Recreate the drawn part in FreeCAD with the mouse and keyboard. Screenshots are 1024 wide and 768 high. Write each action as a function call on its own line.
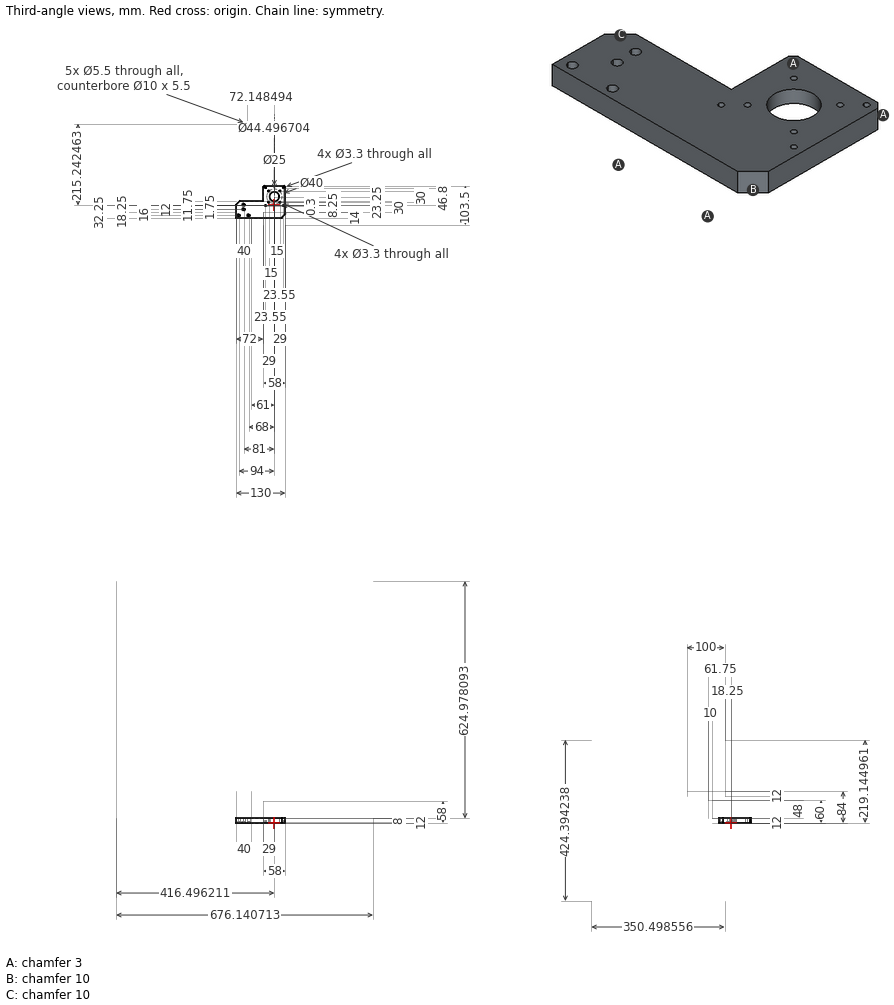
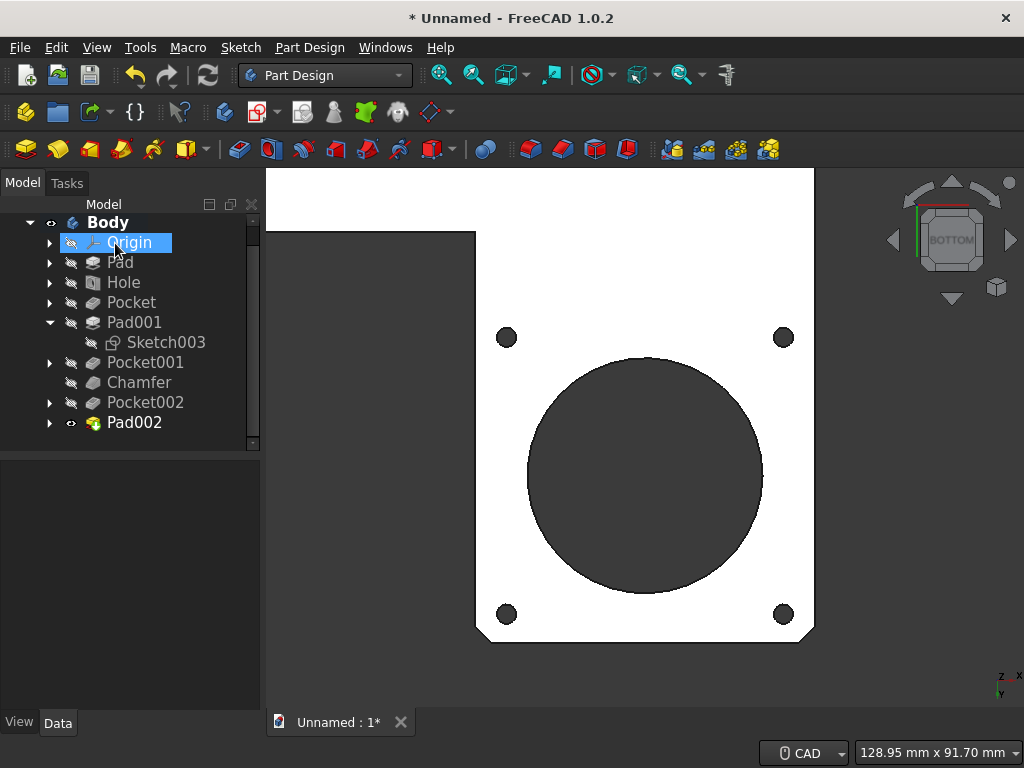
click(442, 76)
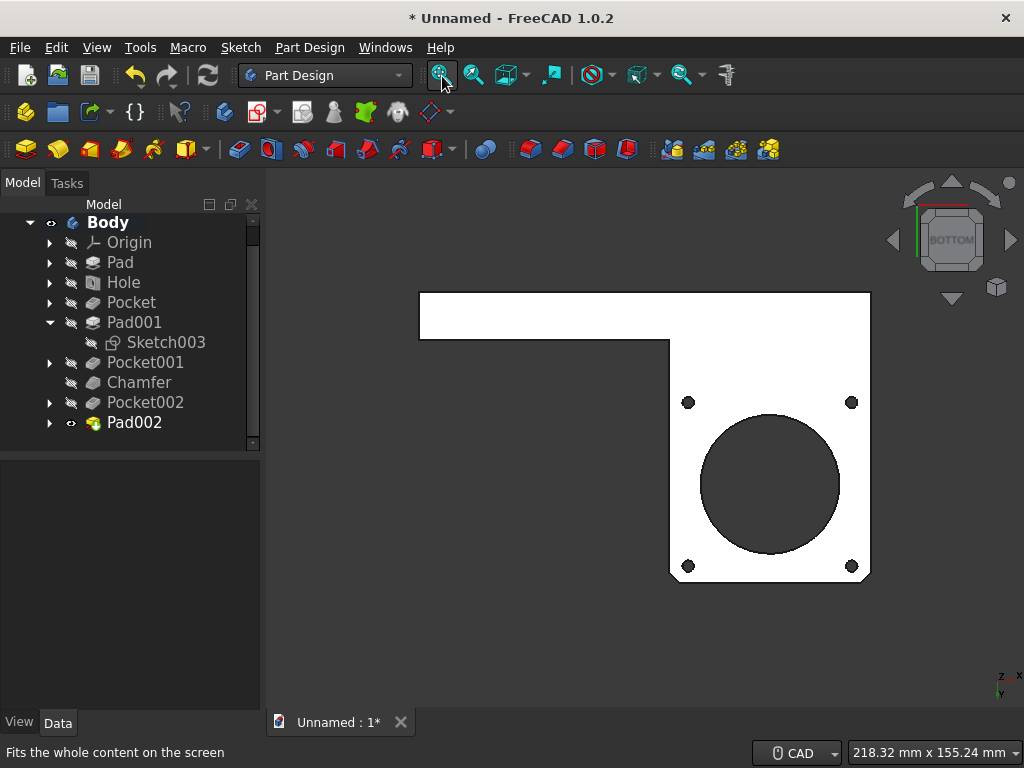
key(0)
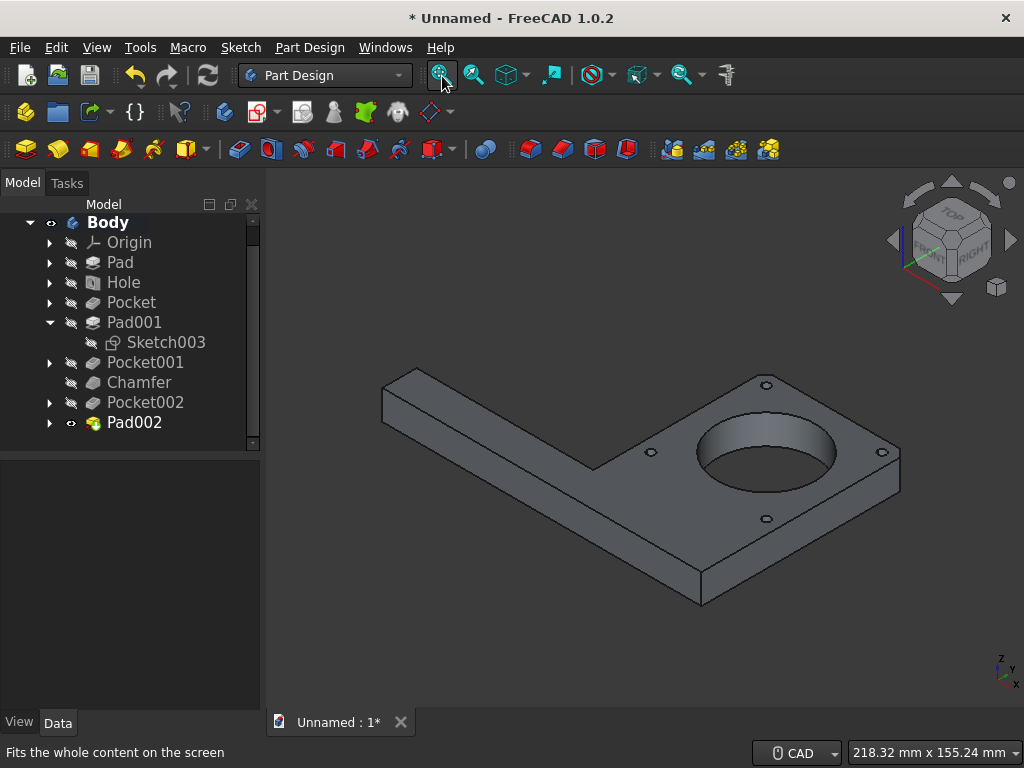
click(677, 506)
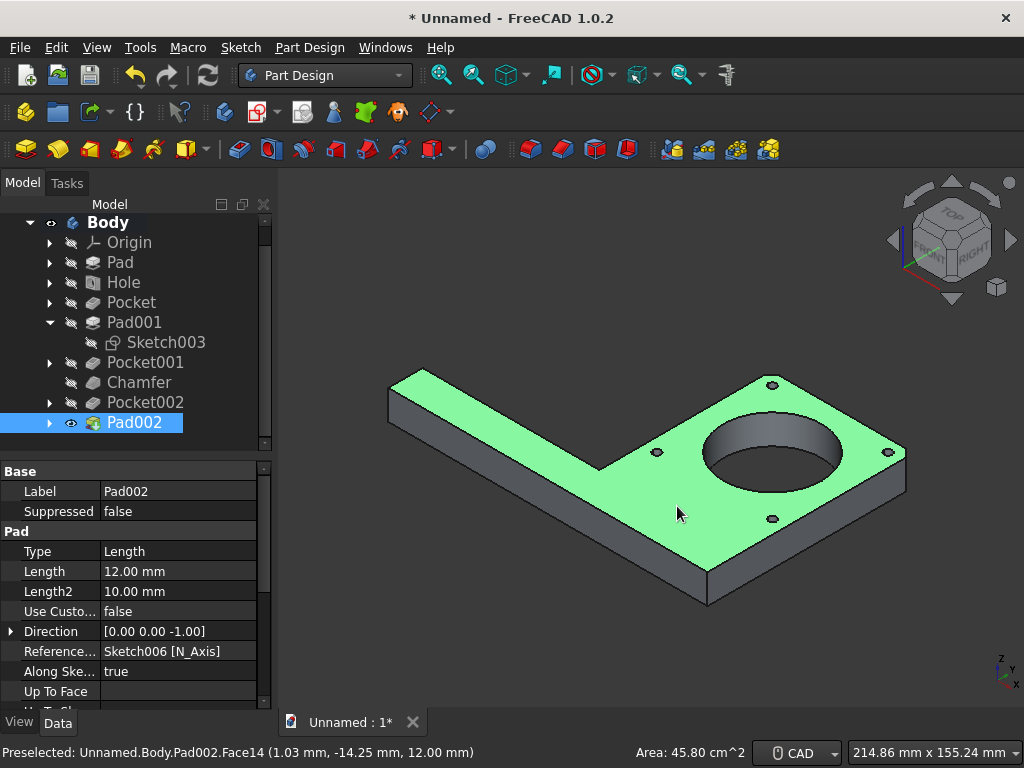
click(258, 112)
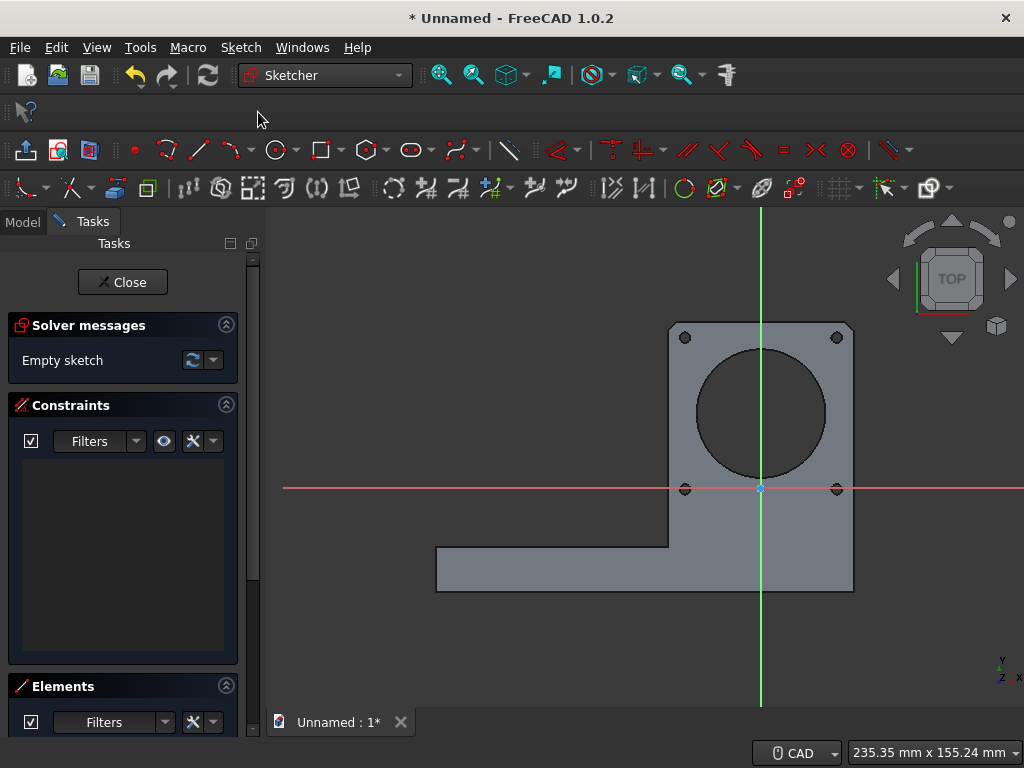
scroll(467, 618, up, 6)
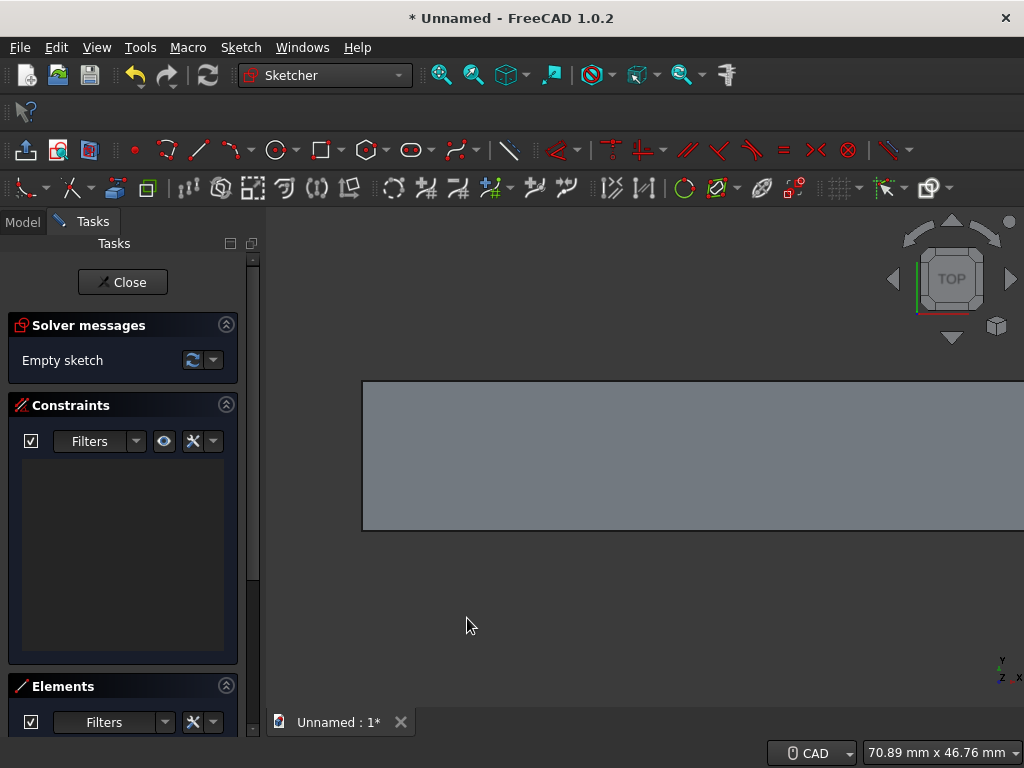
key(g)
key(r)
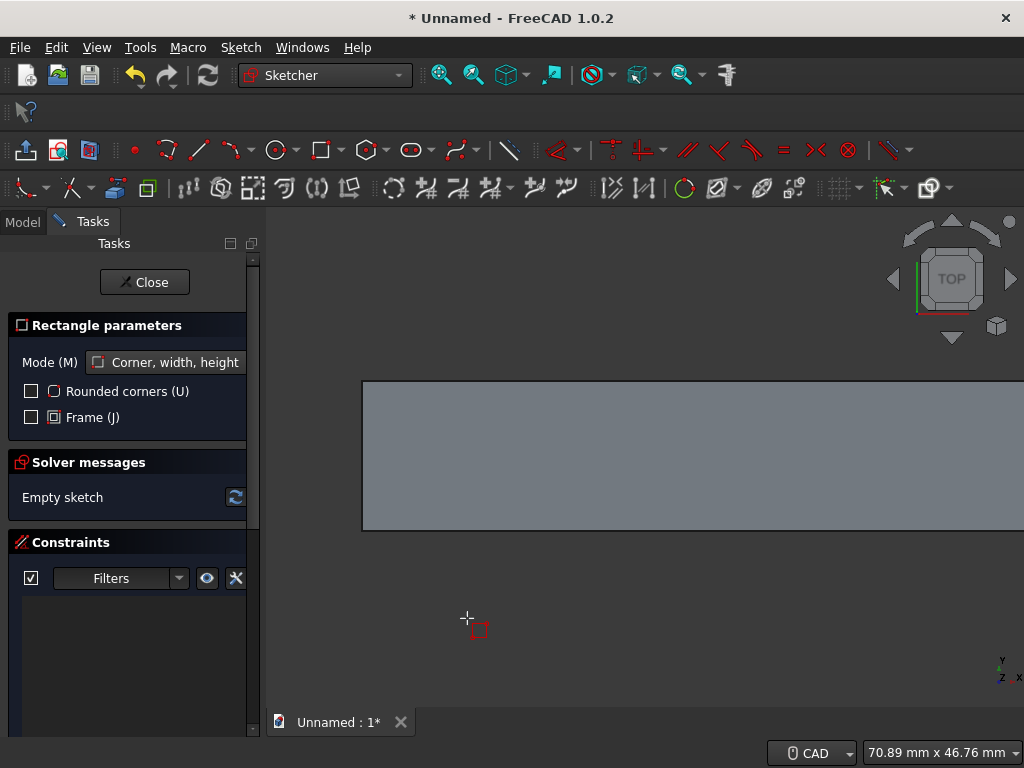
click(362, 381)
move(790, 531)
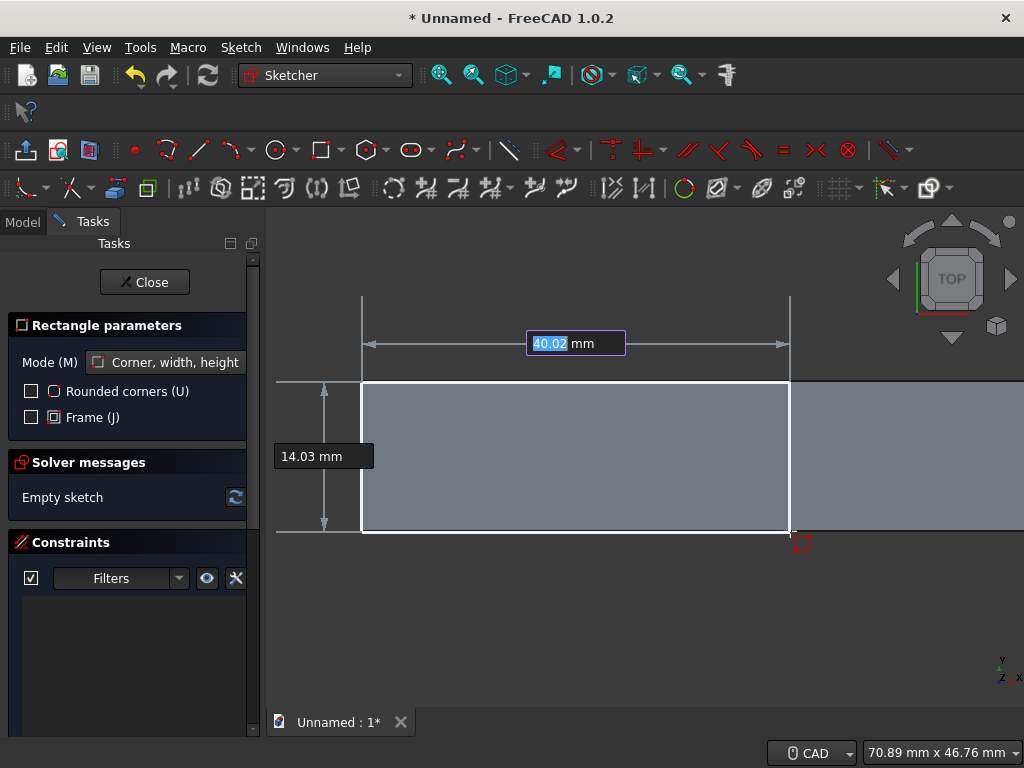
text(40)
key(Tab)
text(14)
key(Return)
key(Escape)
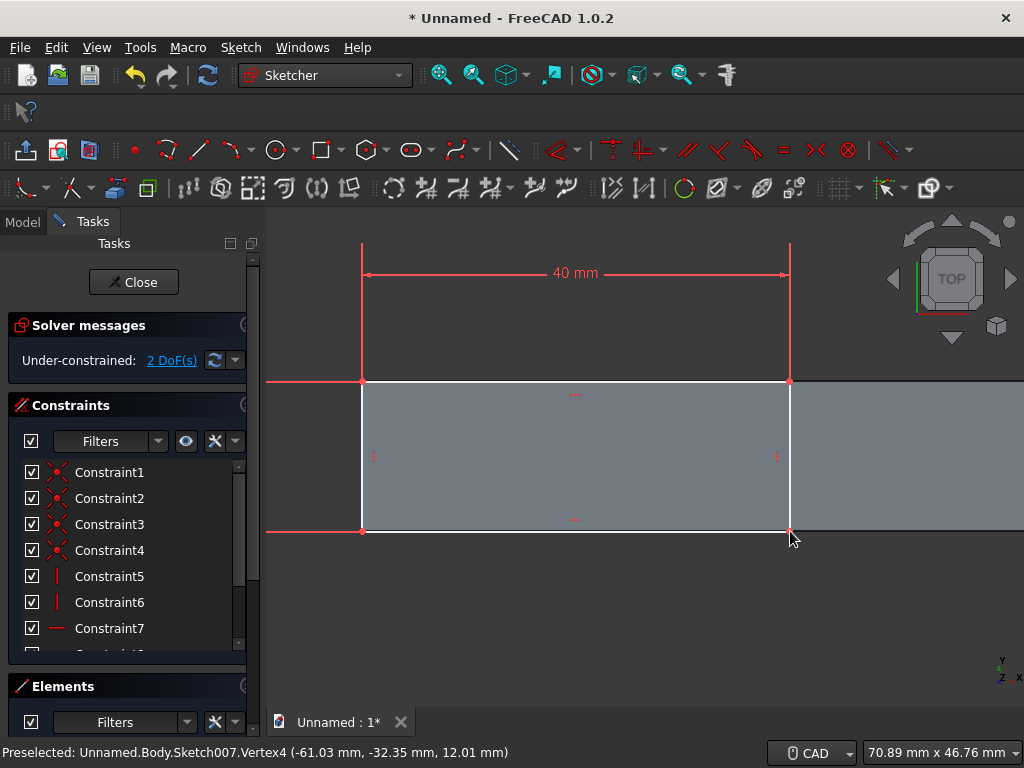
click(556, 150)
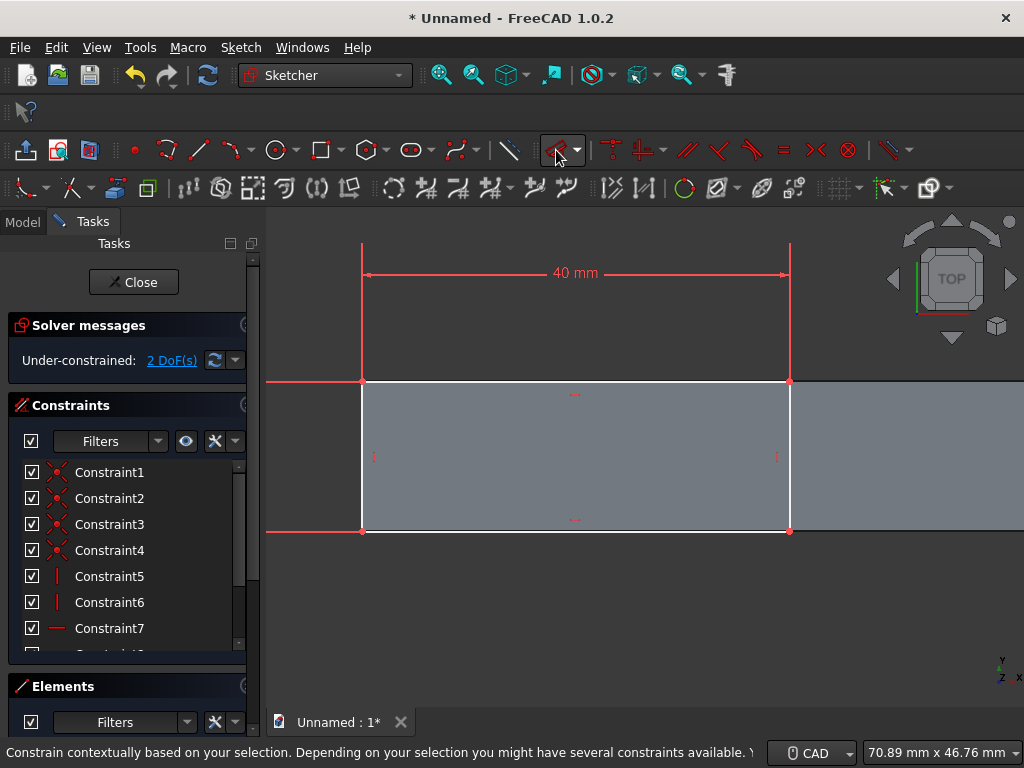
click(790, 532)
click(824, 566)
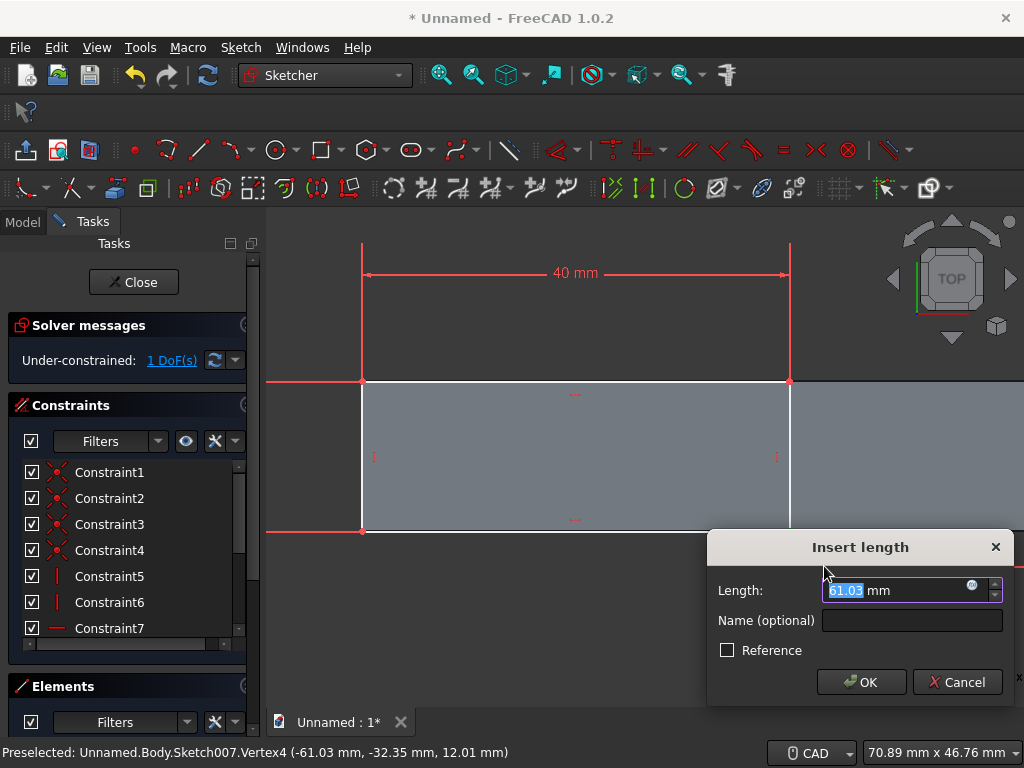
text(61)
key(Return)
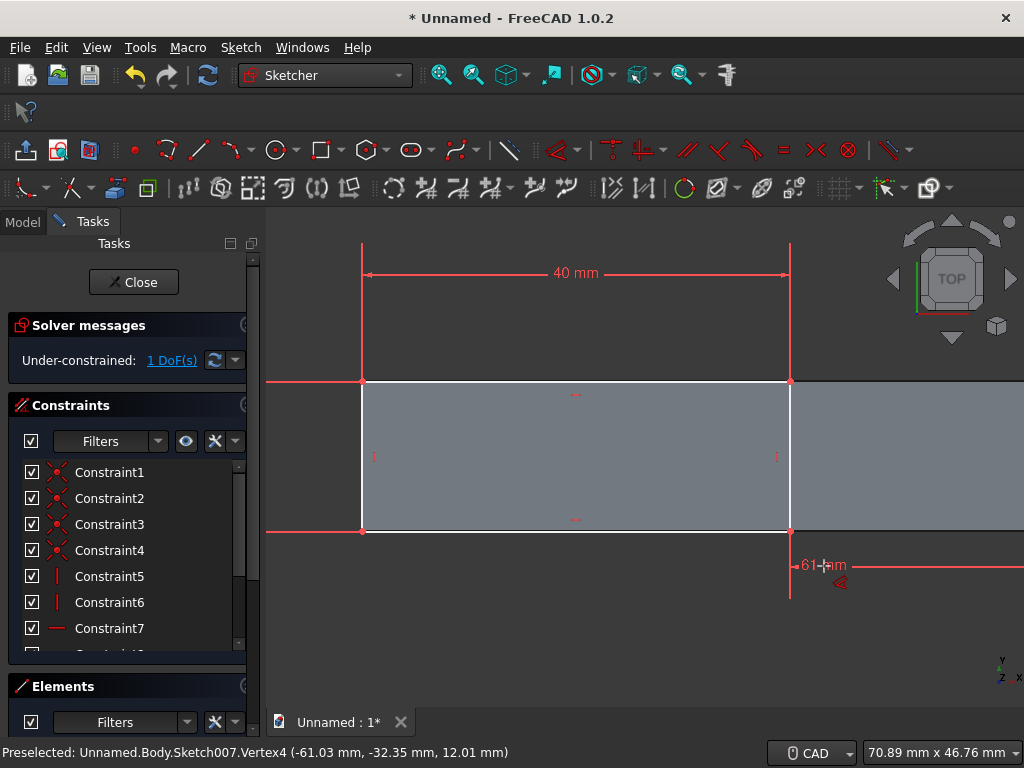
click(362, 382)
click(328, 309)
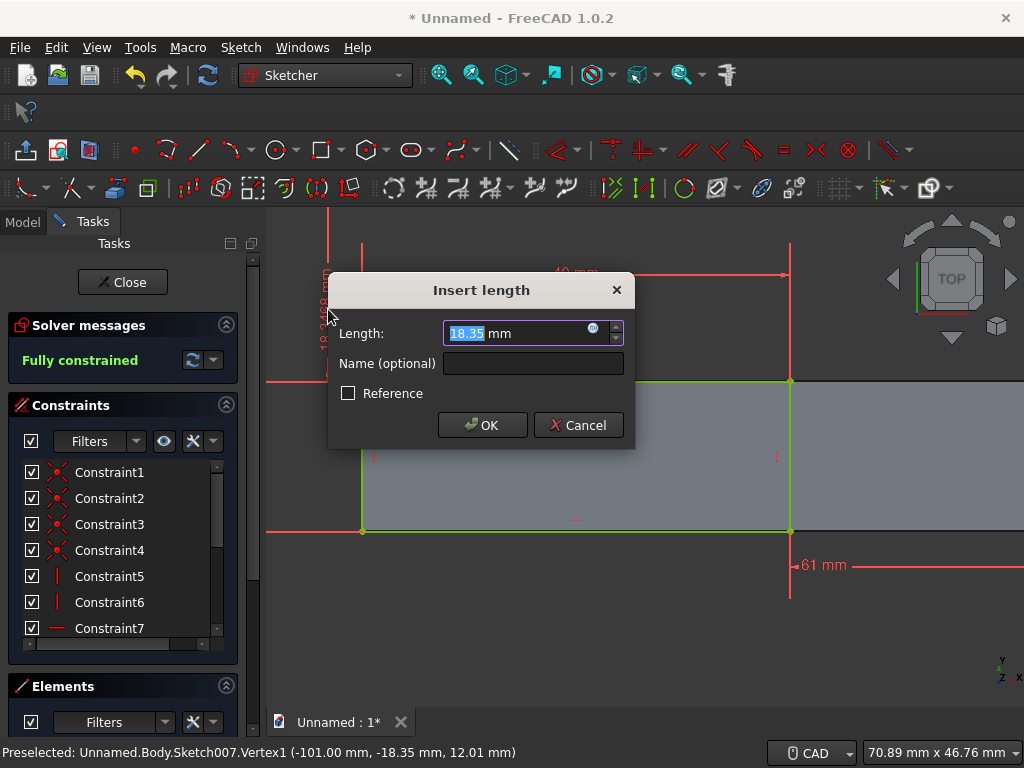
text(18.25)
key(Return)
key(Escape)